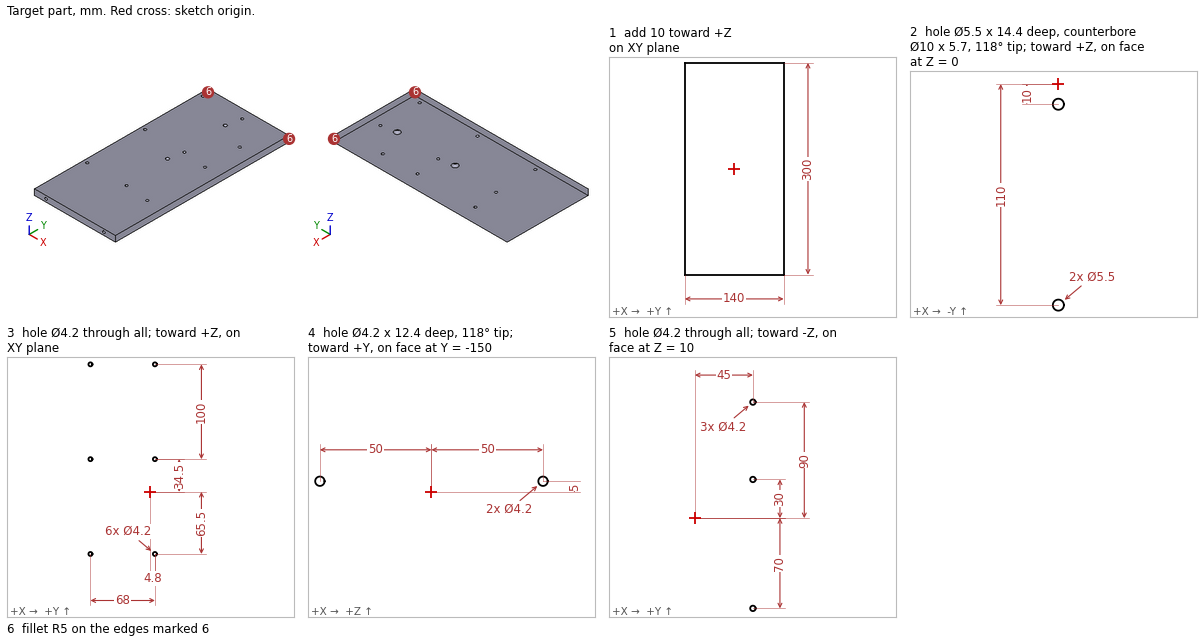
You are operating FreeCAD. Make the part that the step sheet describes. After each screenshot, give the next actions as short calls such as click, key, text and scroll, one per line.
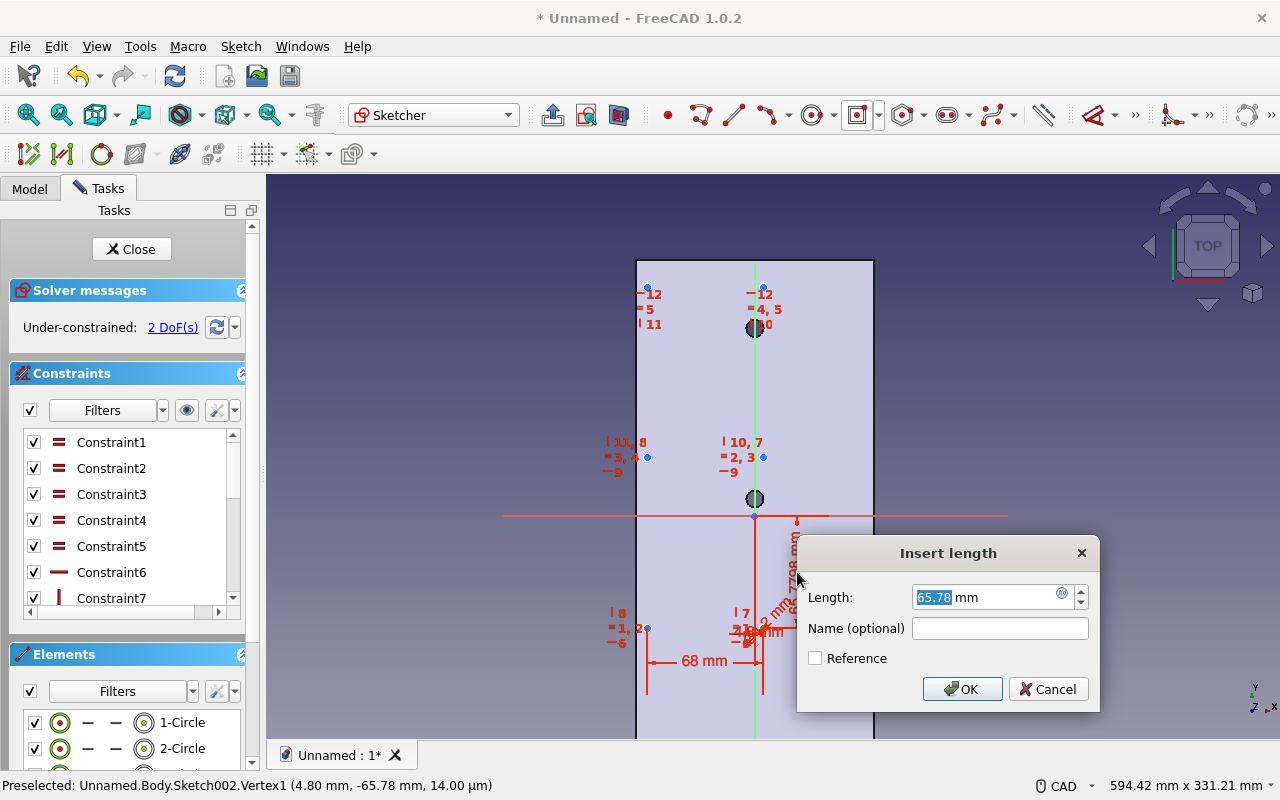
text(65.5)
key(Return)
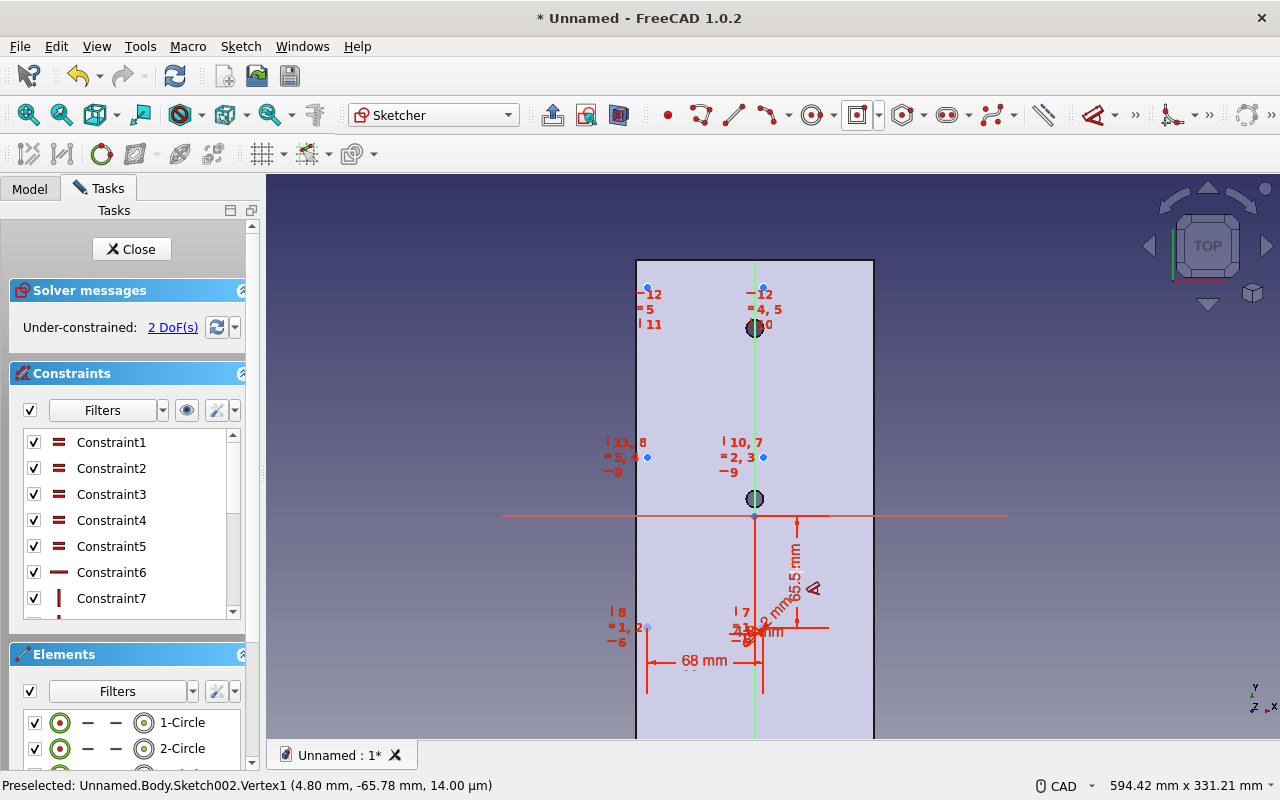
click(763, 458)
click(797, 487)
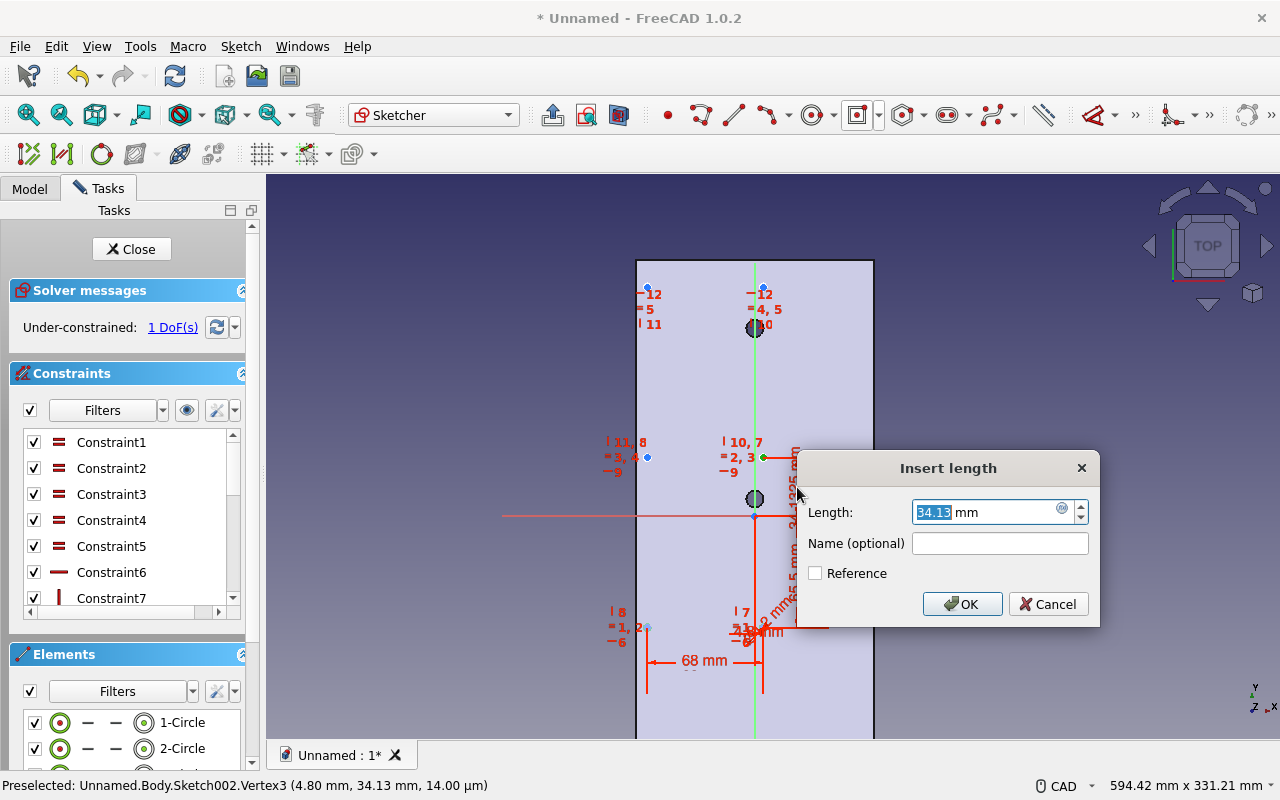
text(34.5)
key(Return)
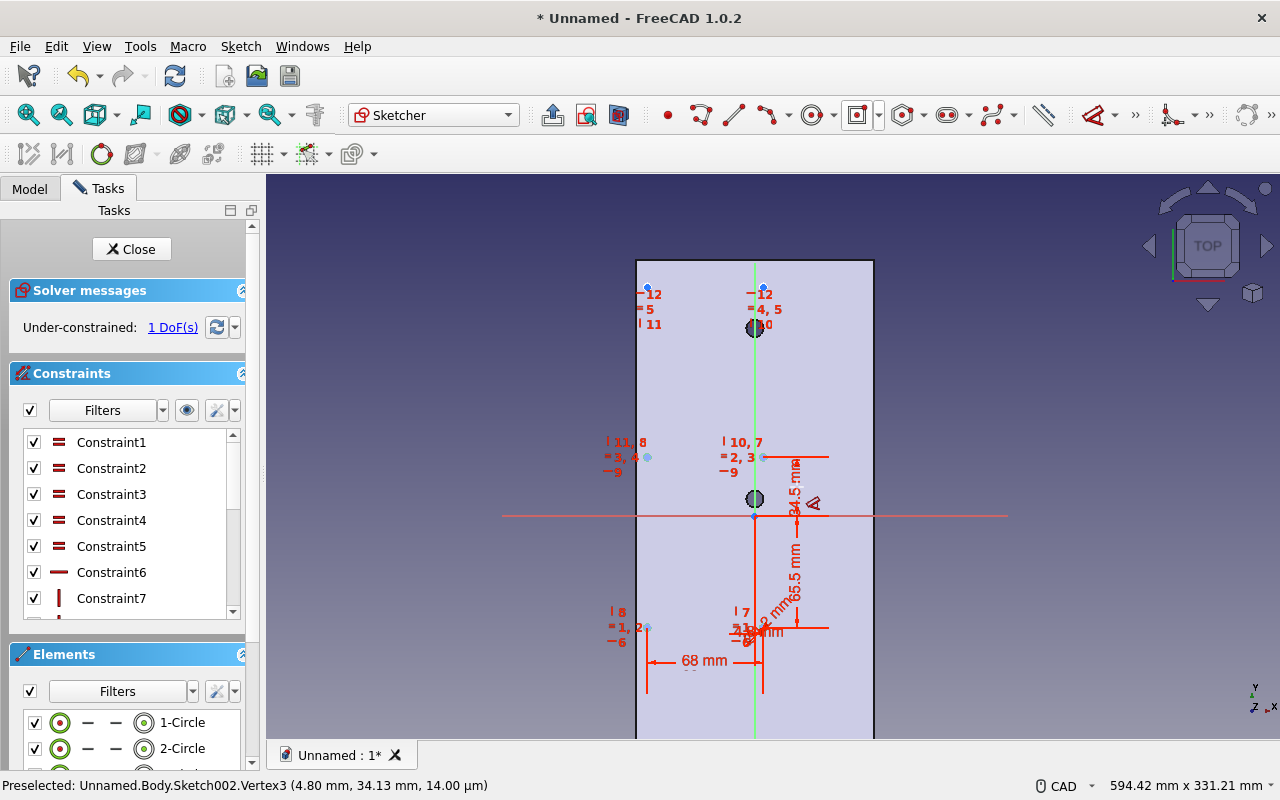
click(763, 457)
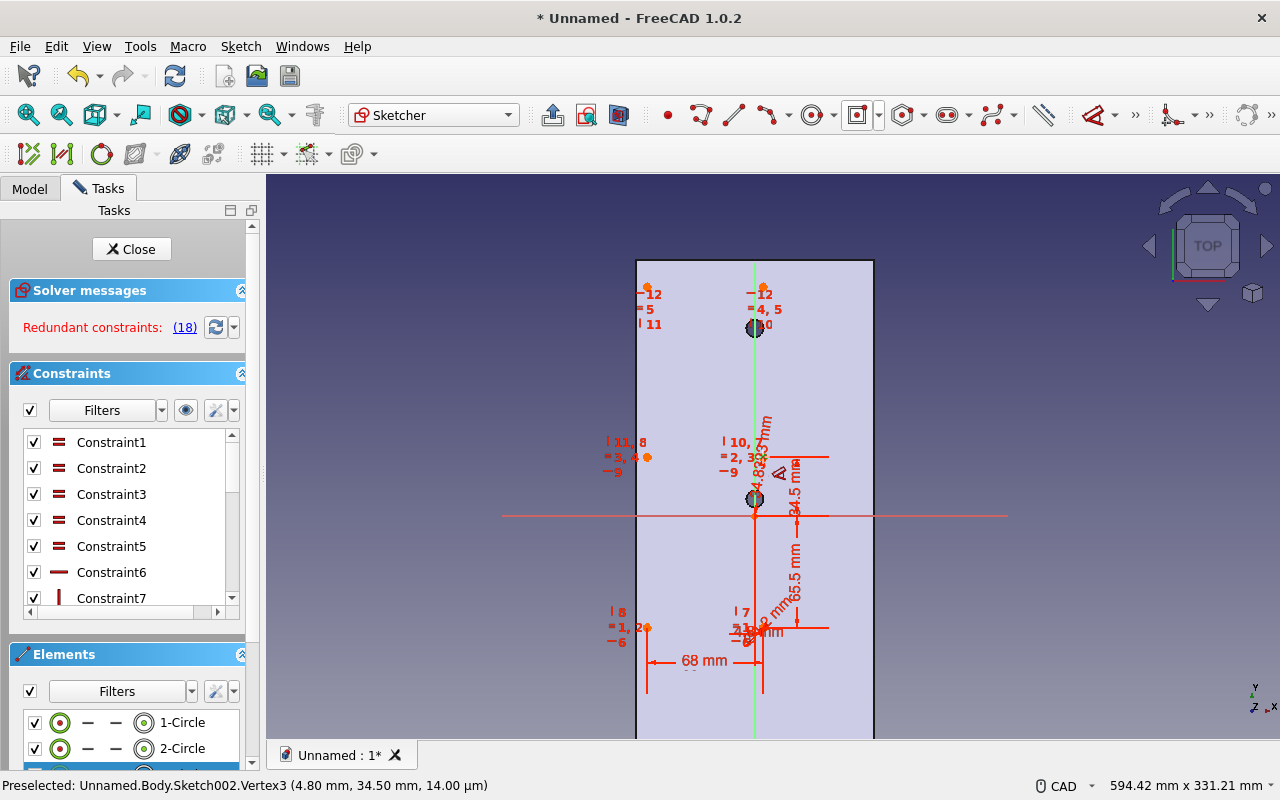
click(763, 287)
click(797, 372)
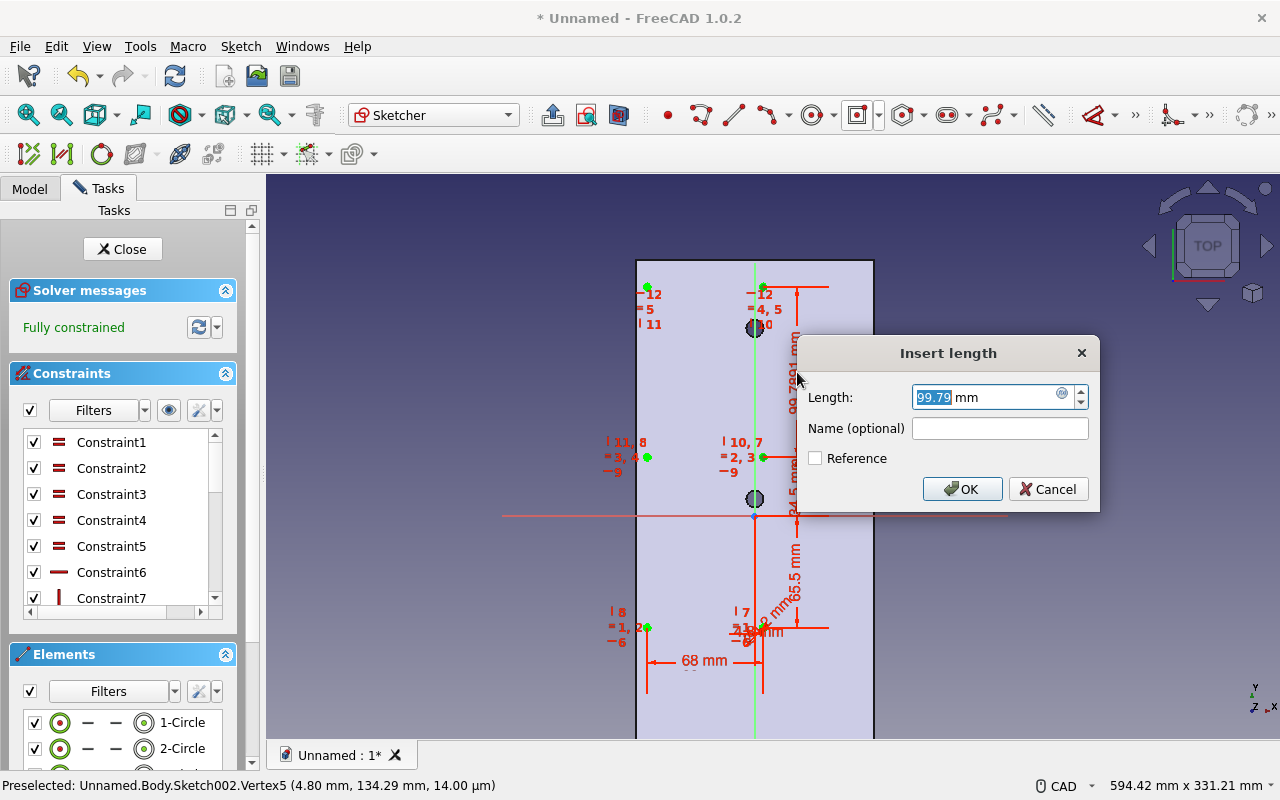
text(100)
key(Return)
key(Escape)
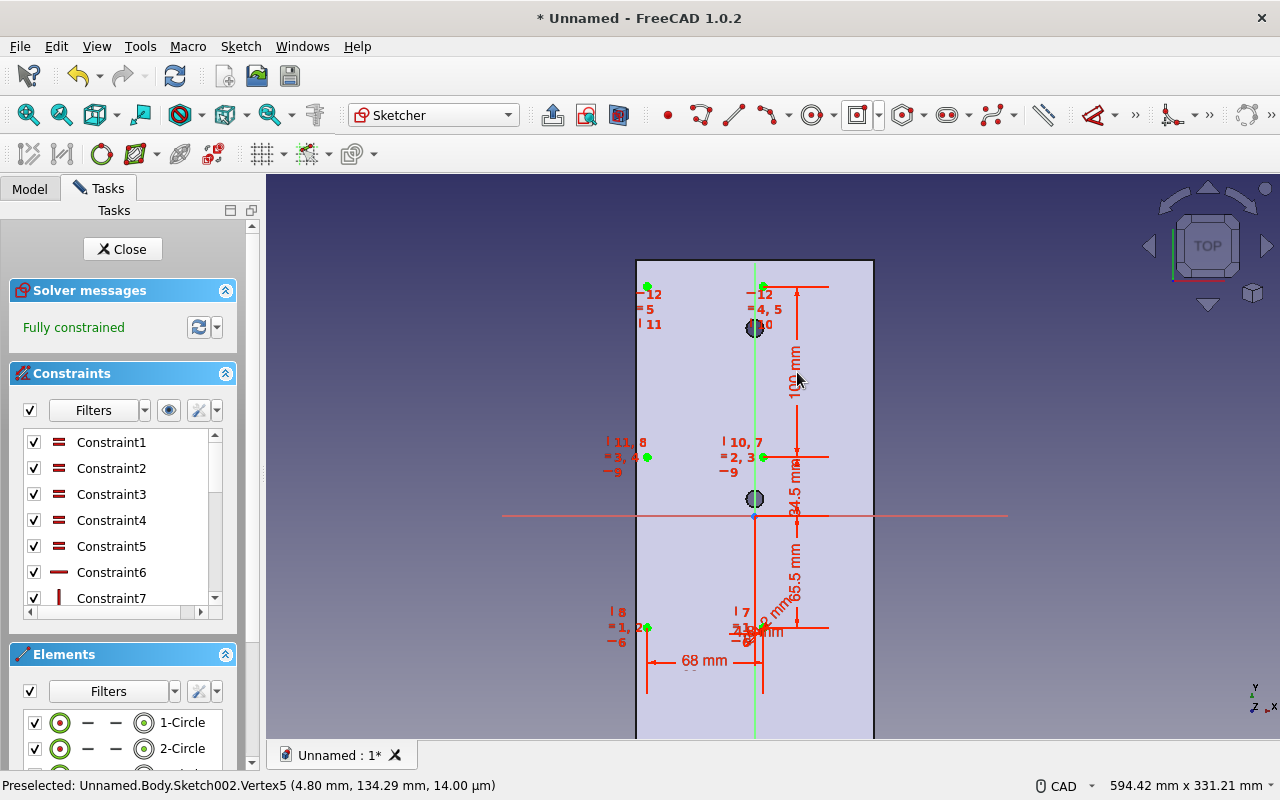
click(123, 249)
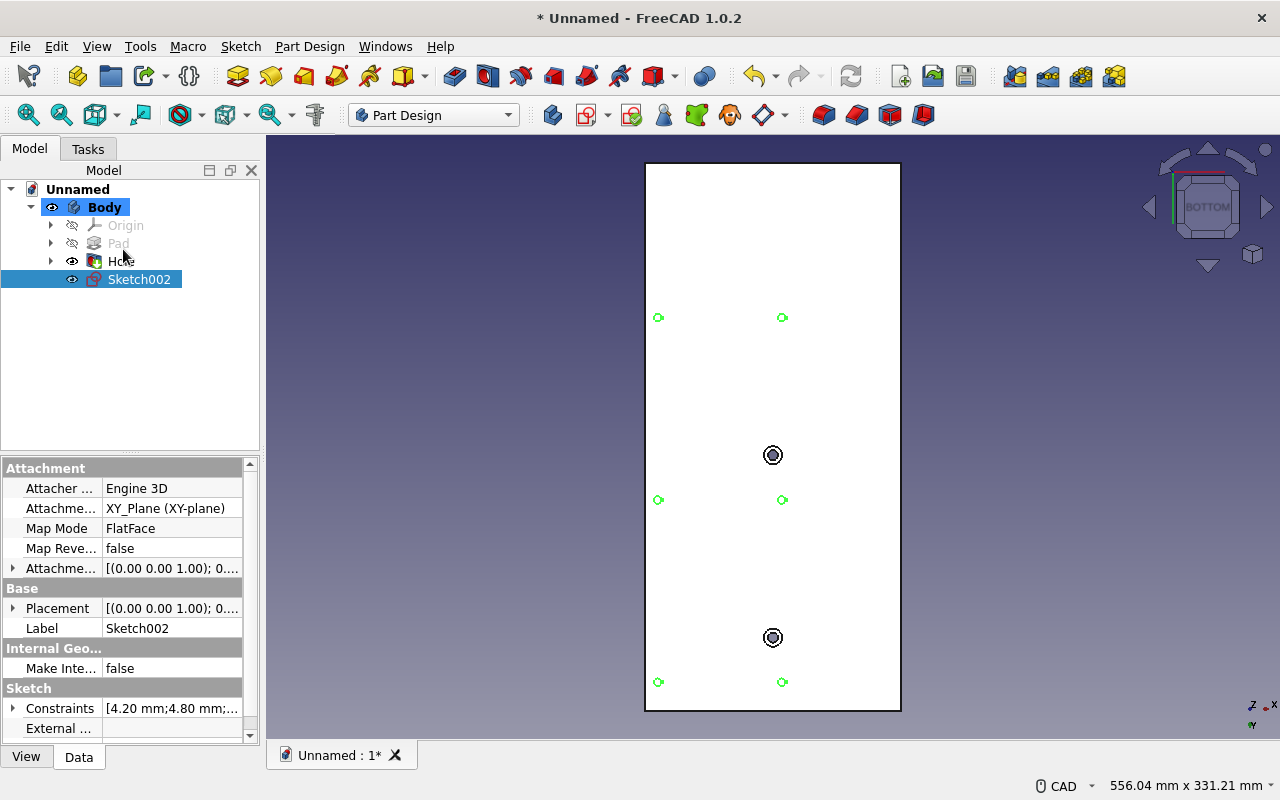
click(488, 76)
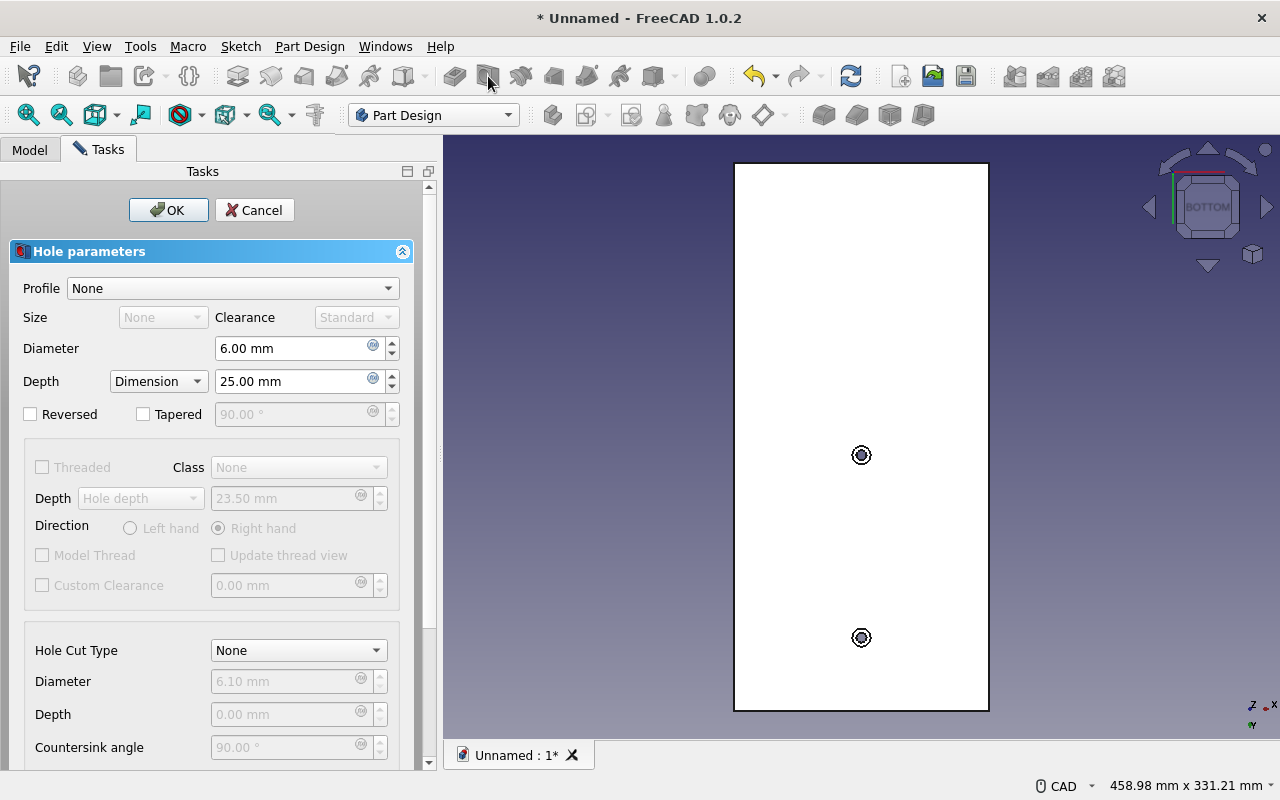
triple_click(300, 348)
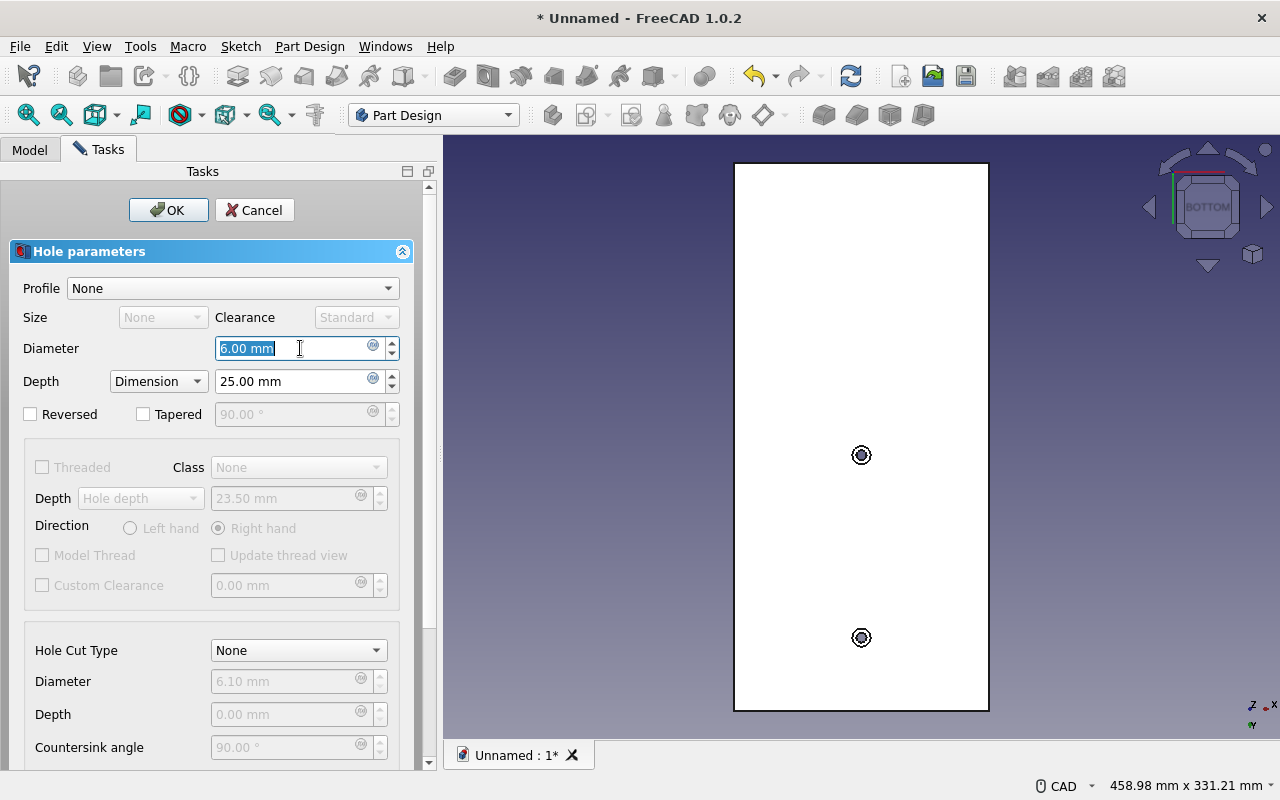
text(4.2)
key(Tab)